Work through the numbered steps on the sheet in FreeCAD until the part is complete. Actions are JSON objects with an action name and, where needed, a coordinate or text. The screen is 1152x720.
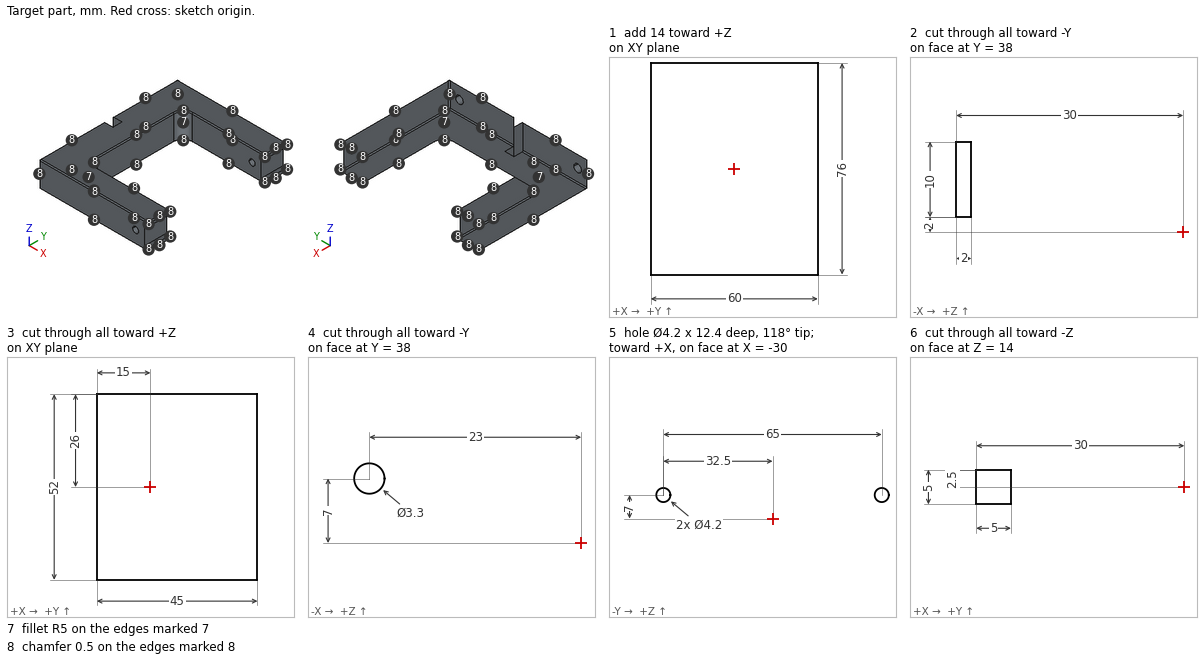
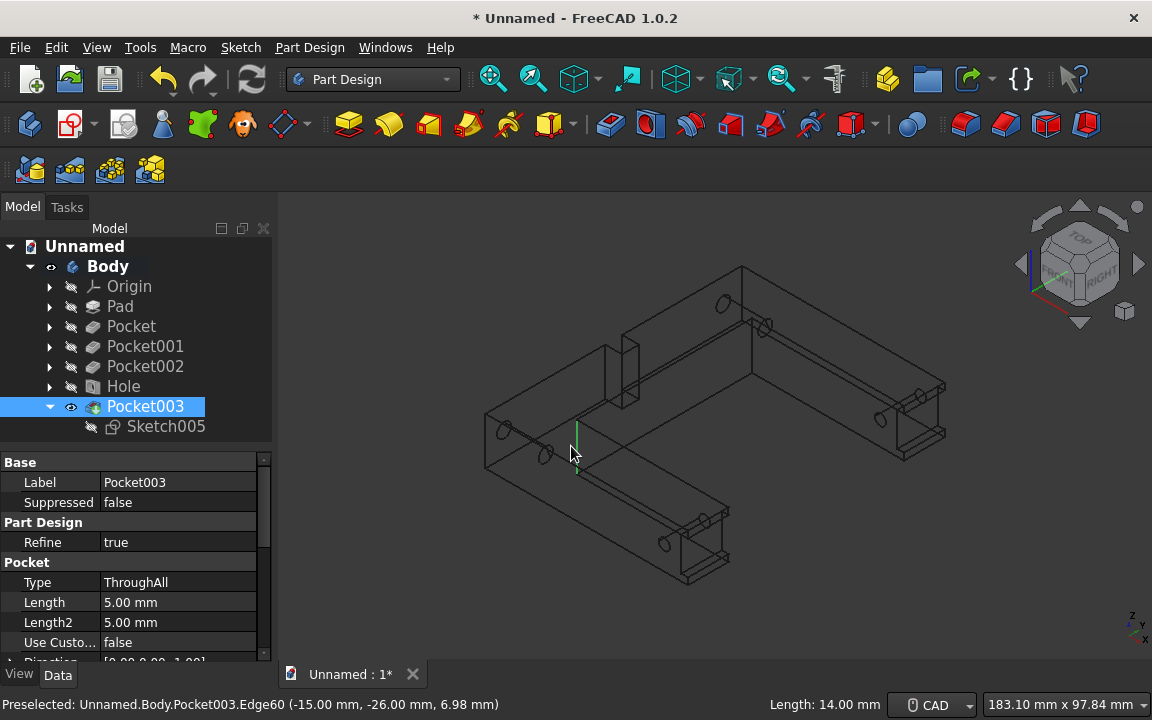
{"action": "left_click", "coordinate": [752, 345], "text": "ctrl"}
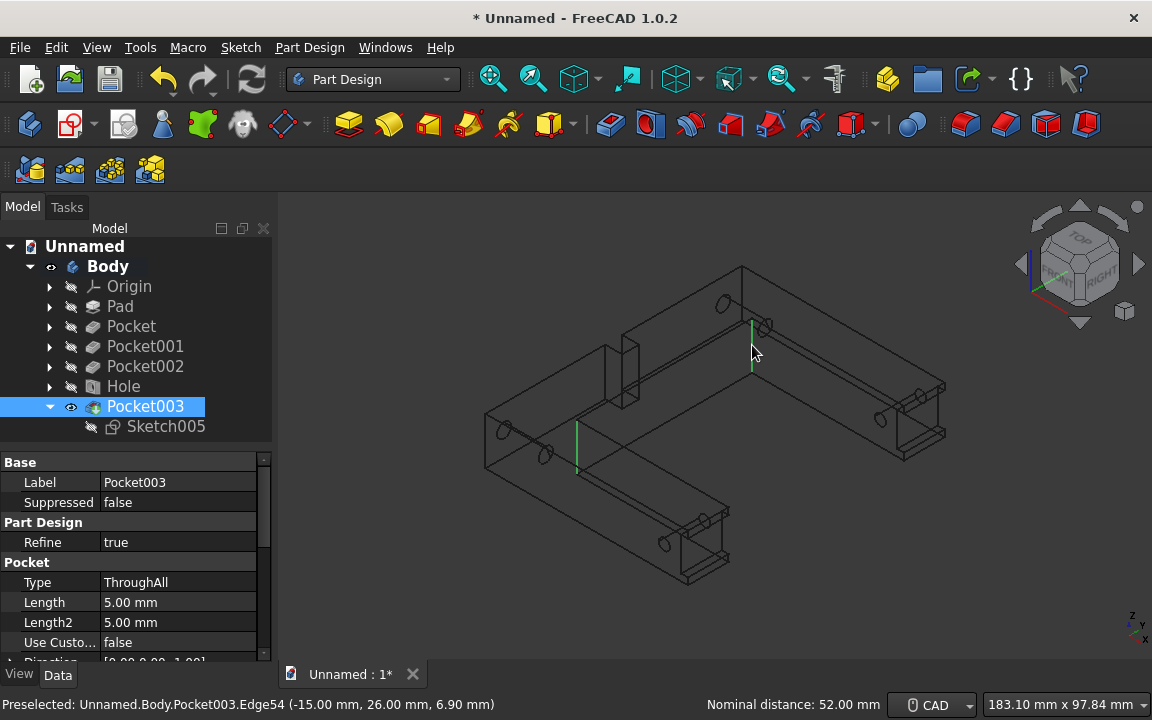
{"action": "key", "text": "v 1"}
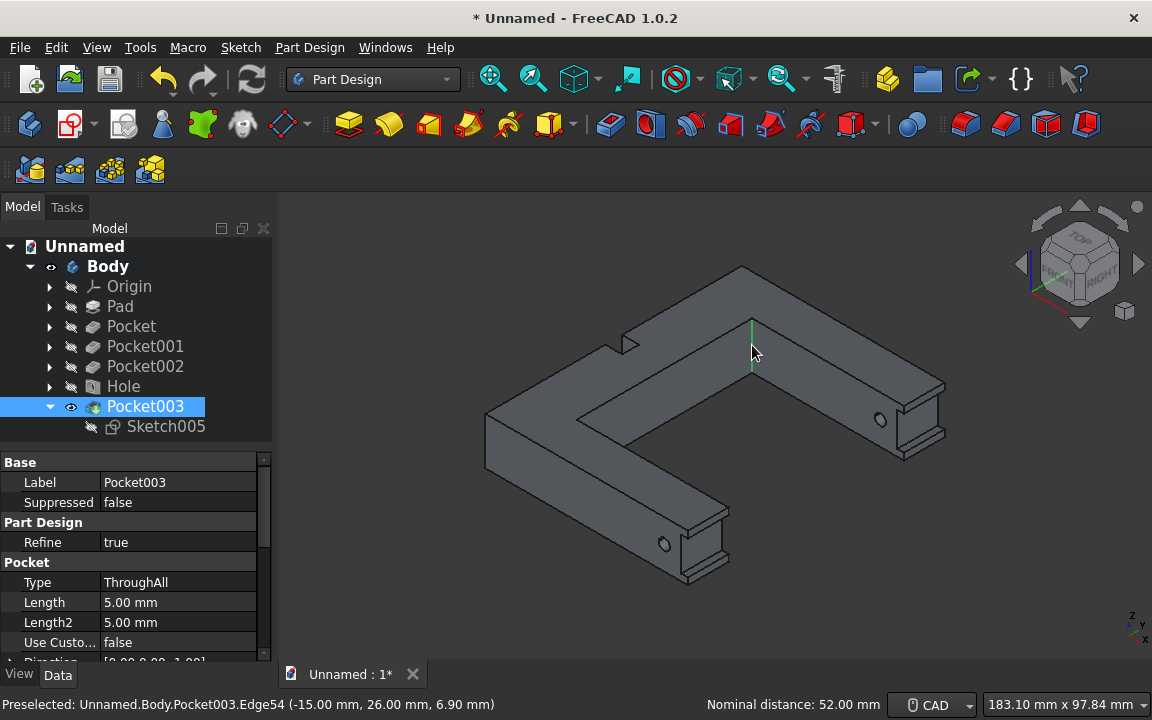
{"action": "left_click", "coordinate": [966, 124]}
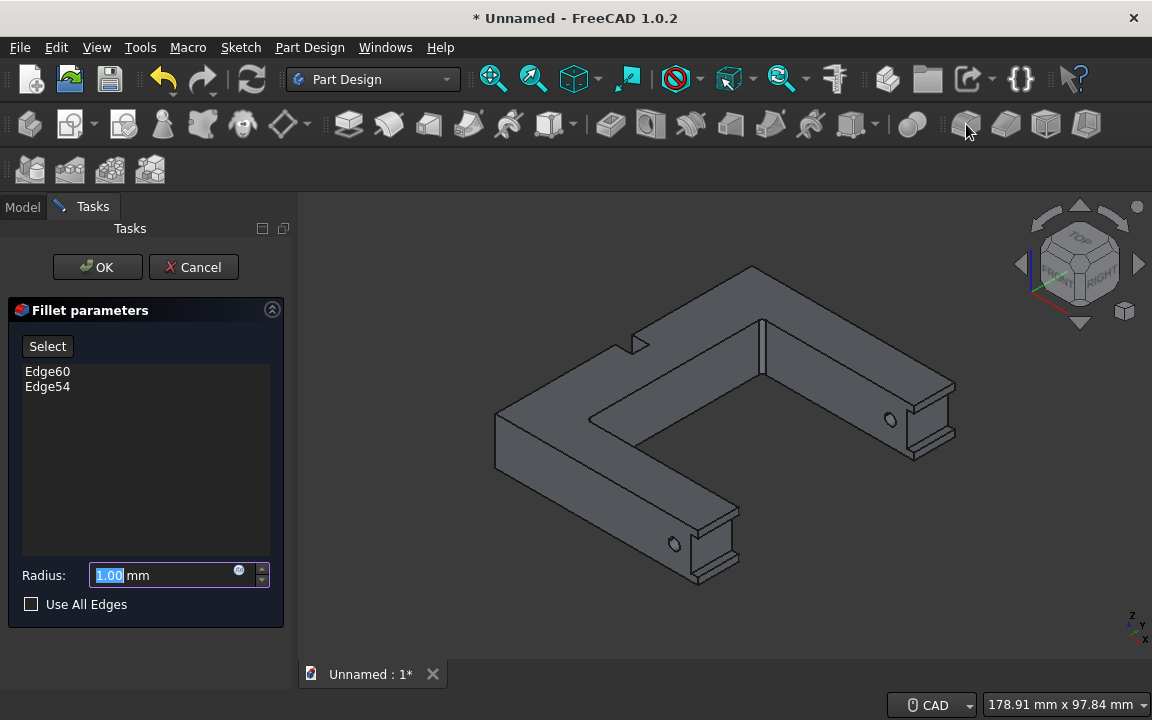
{"action": "type", "text": "5"}
{"action": "key", "text": "Tab"}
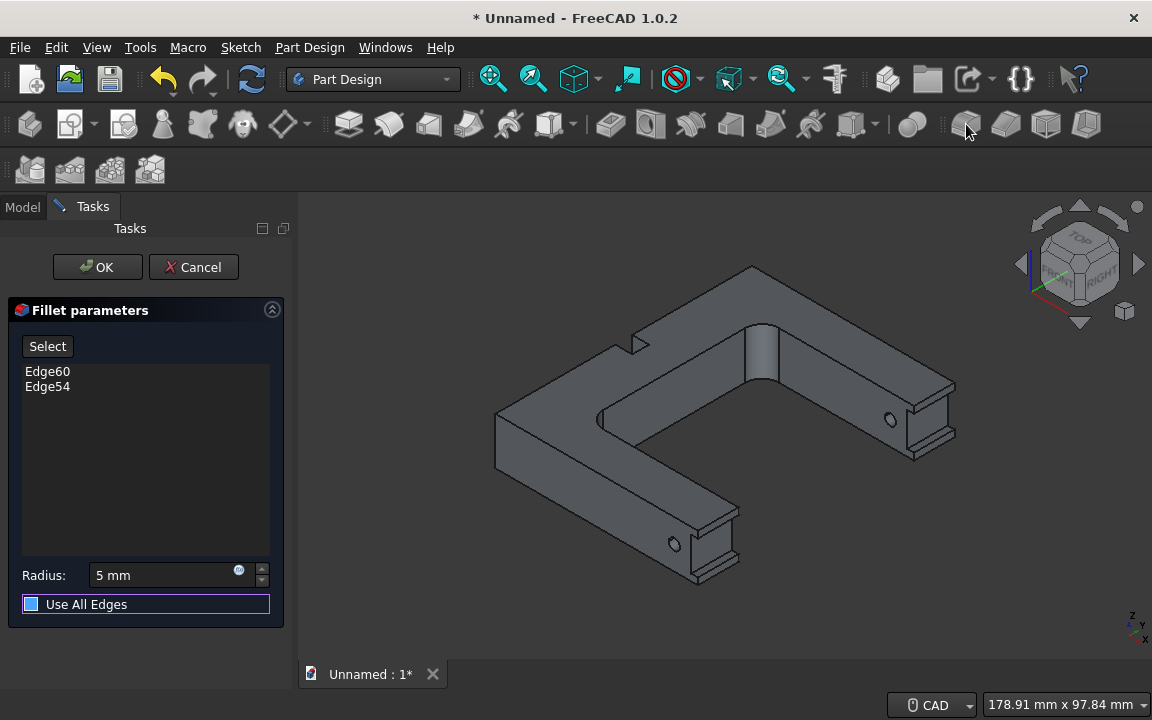
{"action": "left_click", "coordinate": [98, 267]}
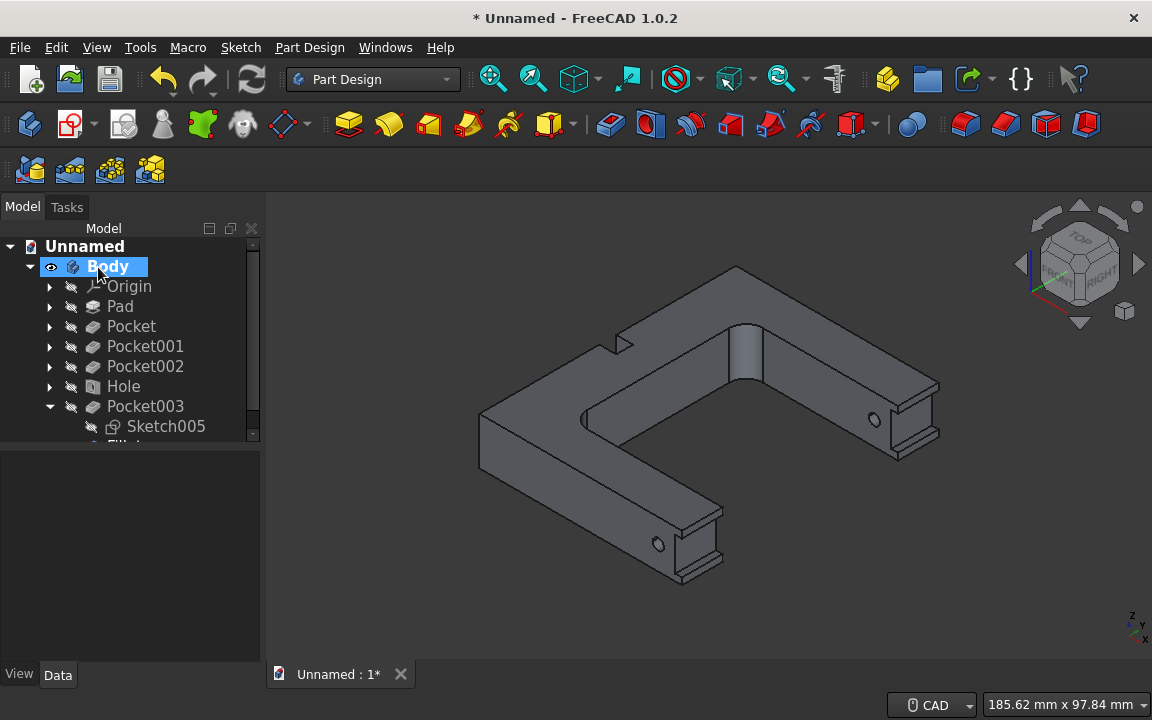
{"action": "left_click", "coordinate": [581, 471]}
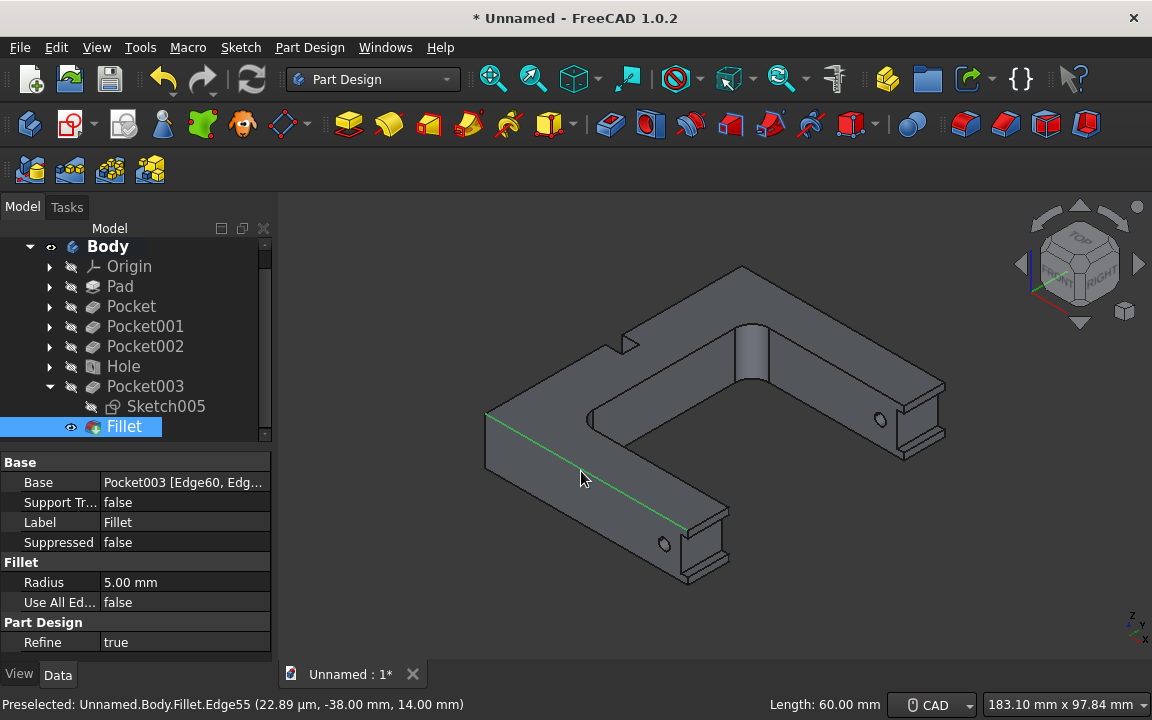
{"action": "left_click", "coordinate": [924, 393], "text": "ctrl"}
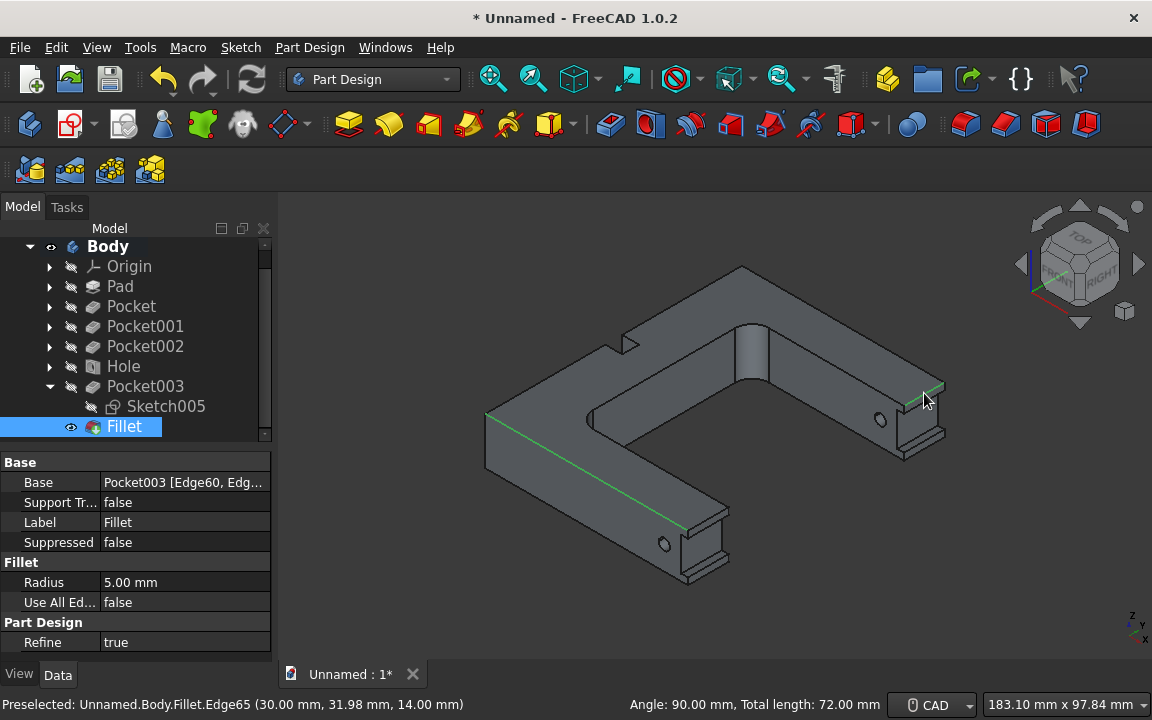
{"action": "left_click", "coordinate": [904, 411], "text": "ctrl"}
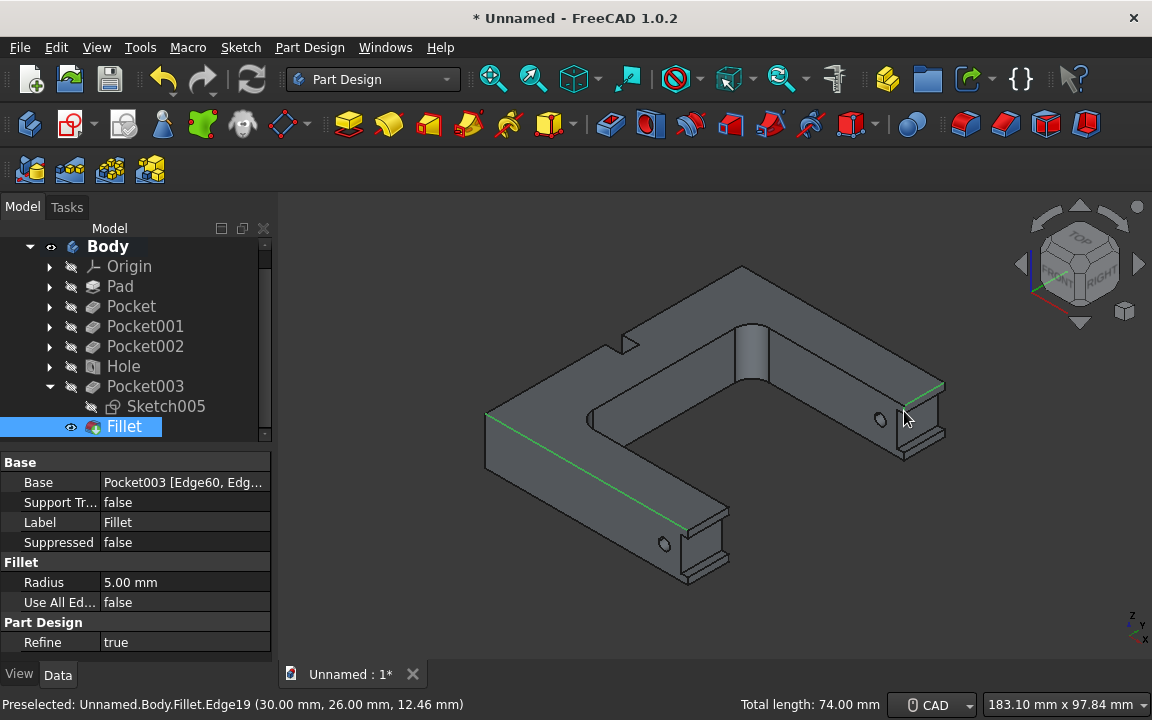
{"action": "left_click", "coordinate": [708, 518], "text": "ctrl"}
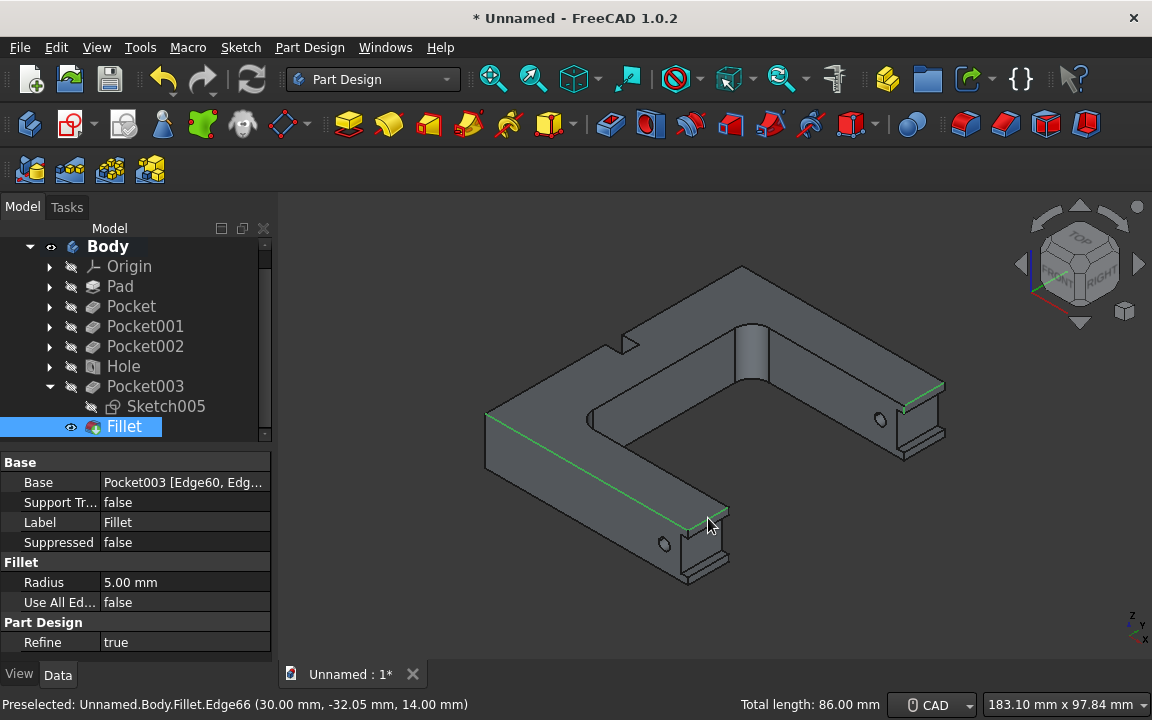
{"action": "left_click", "coordinate": [837, 366], "text": "ctrl"}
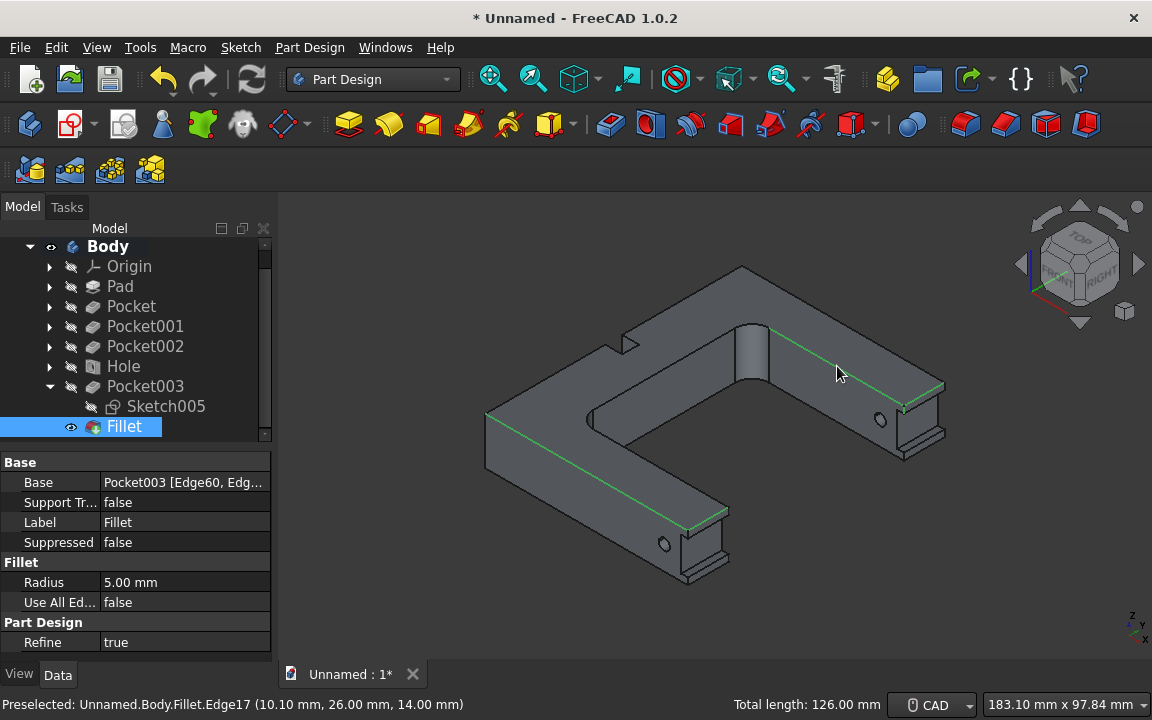
{"action": "left_click", "coordinate": [664, 368], "text": "ctrl"}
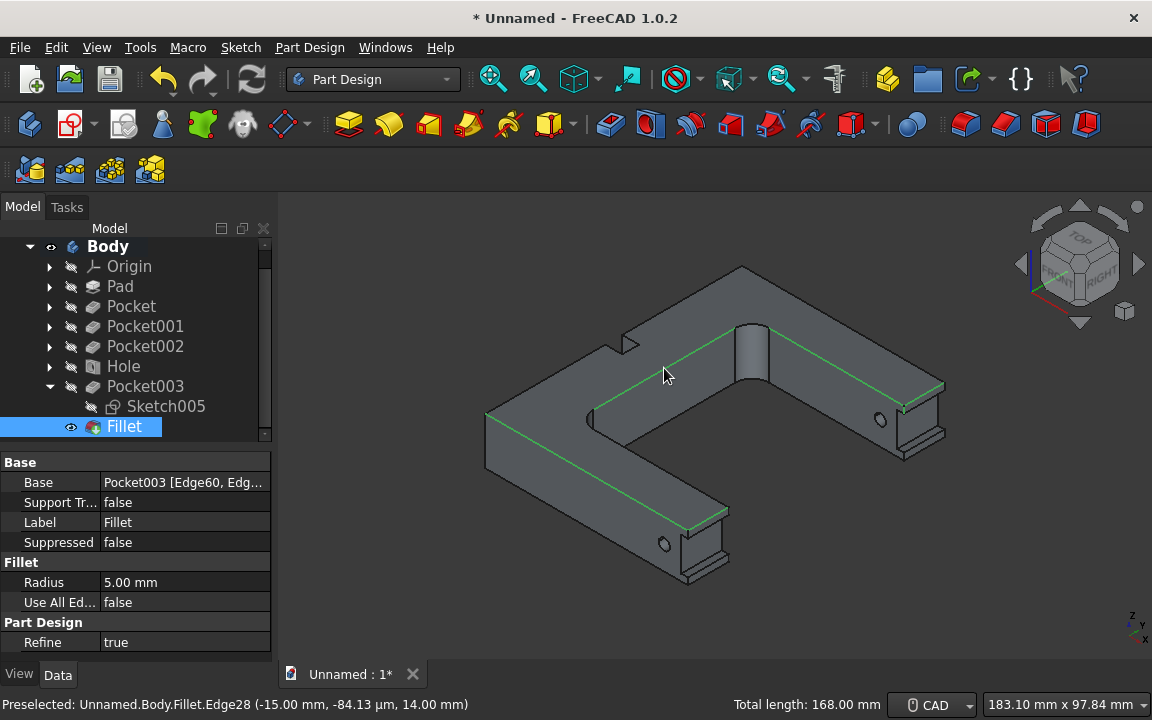
{"action": "left_click", "coordinate": [752, 323], "text": "ctrl"}